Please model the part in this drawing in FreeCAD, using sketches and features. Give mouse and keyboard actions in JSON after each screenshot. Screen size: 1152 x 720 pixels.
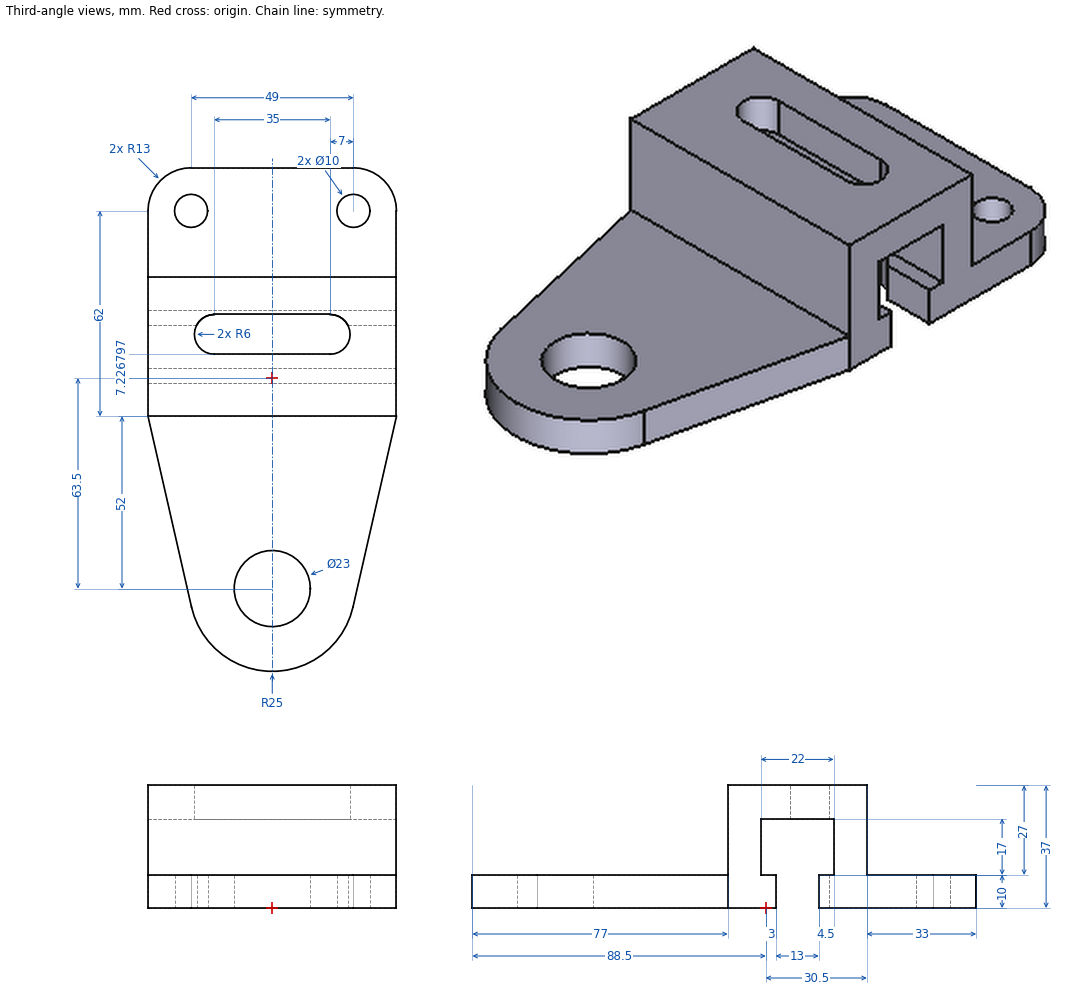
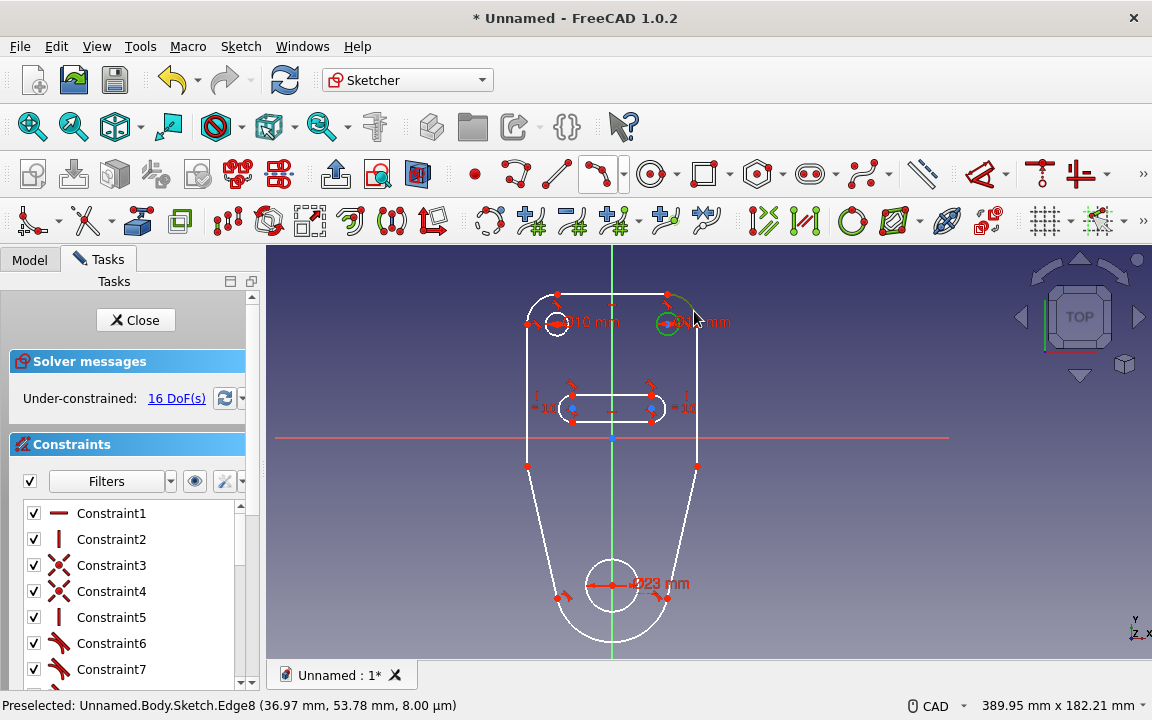
{"action": "left_click", "coordinate": [1040, 174]}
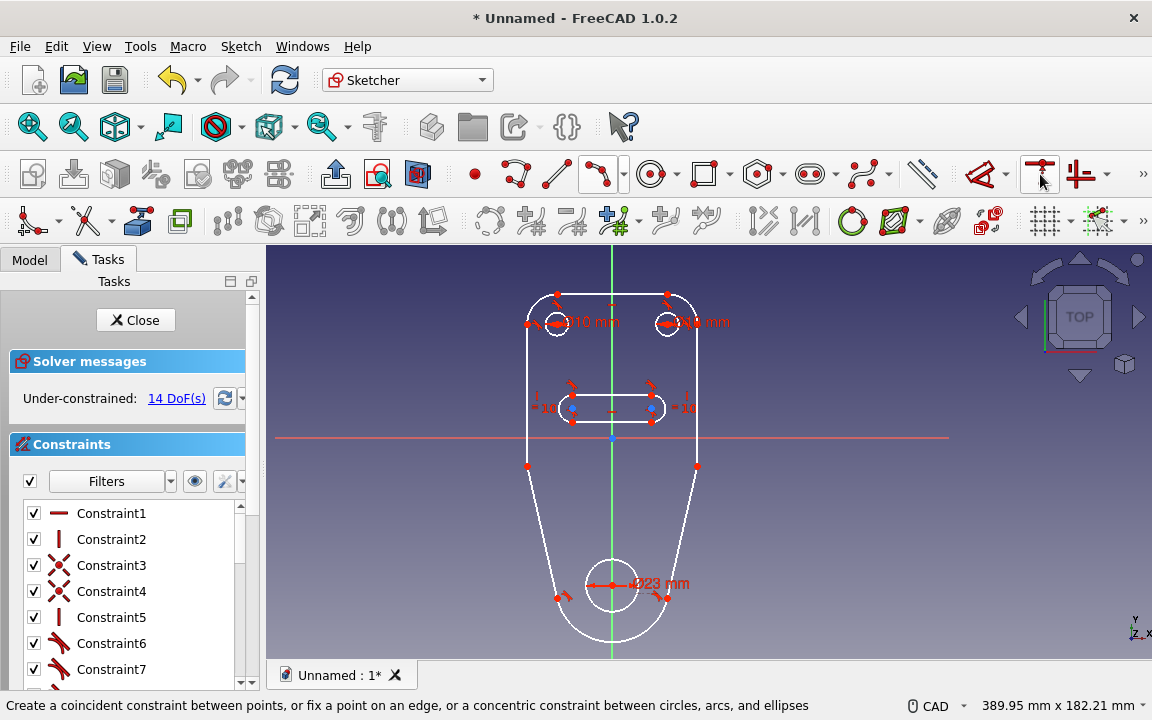
{"action": "left_click", "coordinate": [543, 298]}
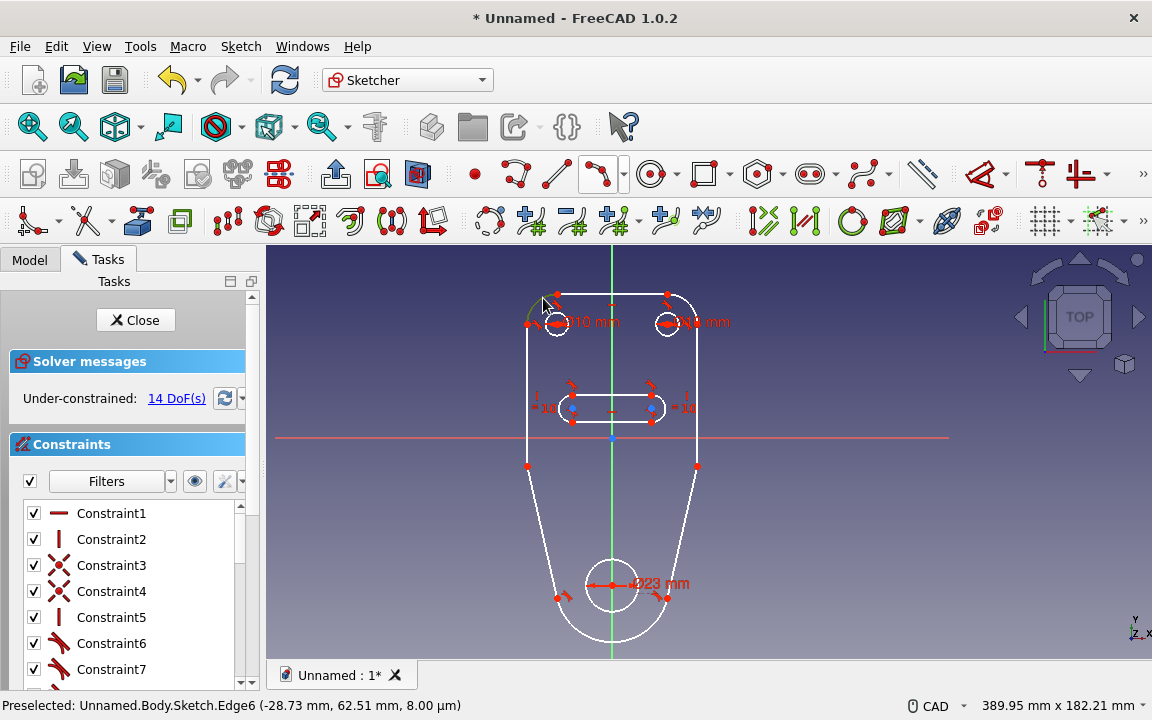
{"action": "left_click", "coordinate": [694, 311]}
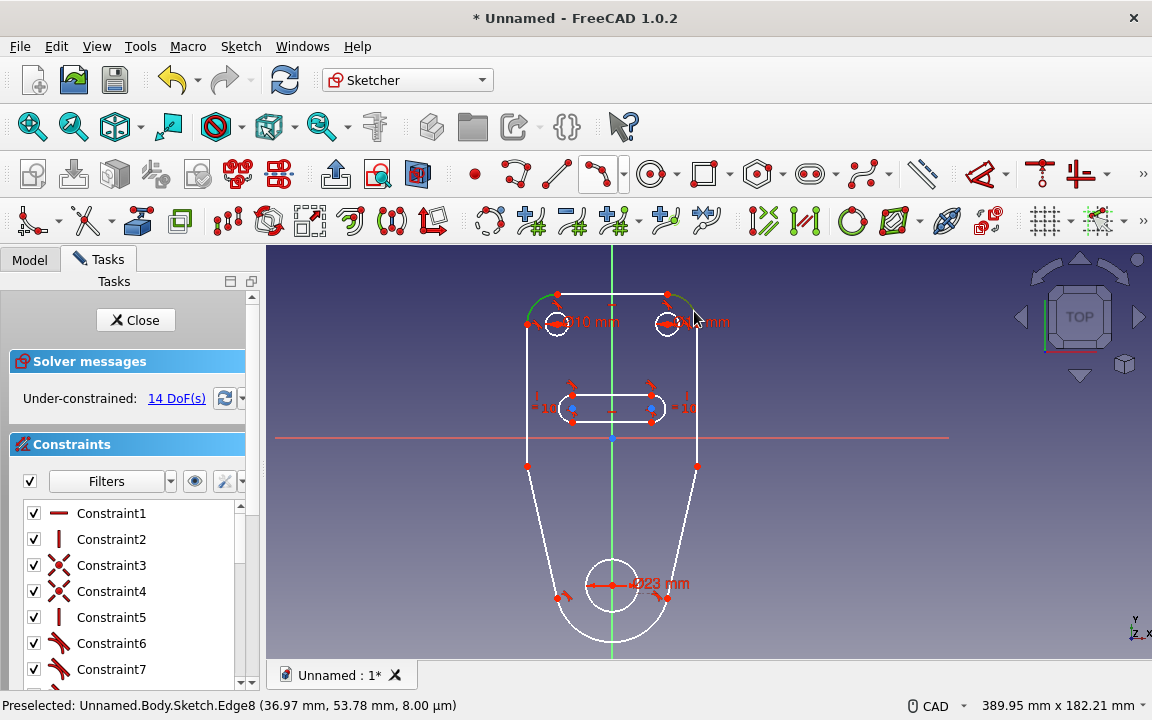
{"action": "key", "text": "e"}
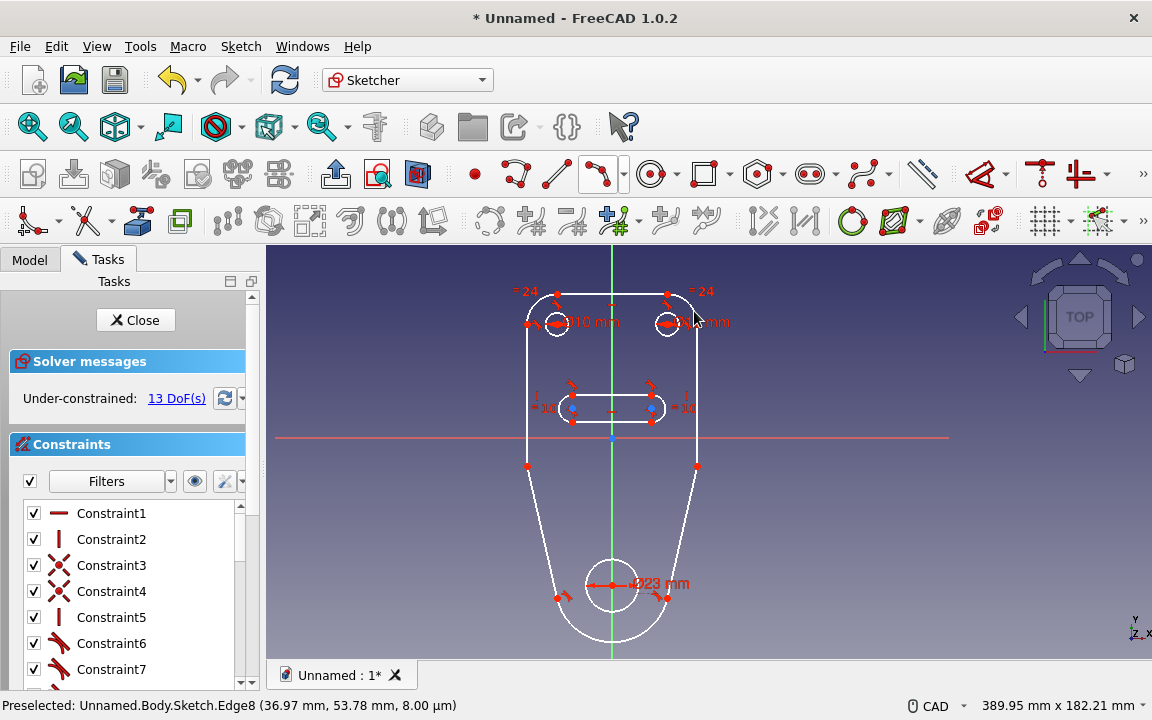
{"action": "left_click", "coordinate": [612, 586]}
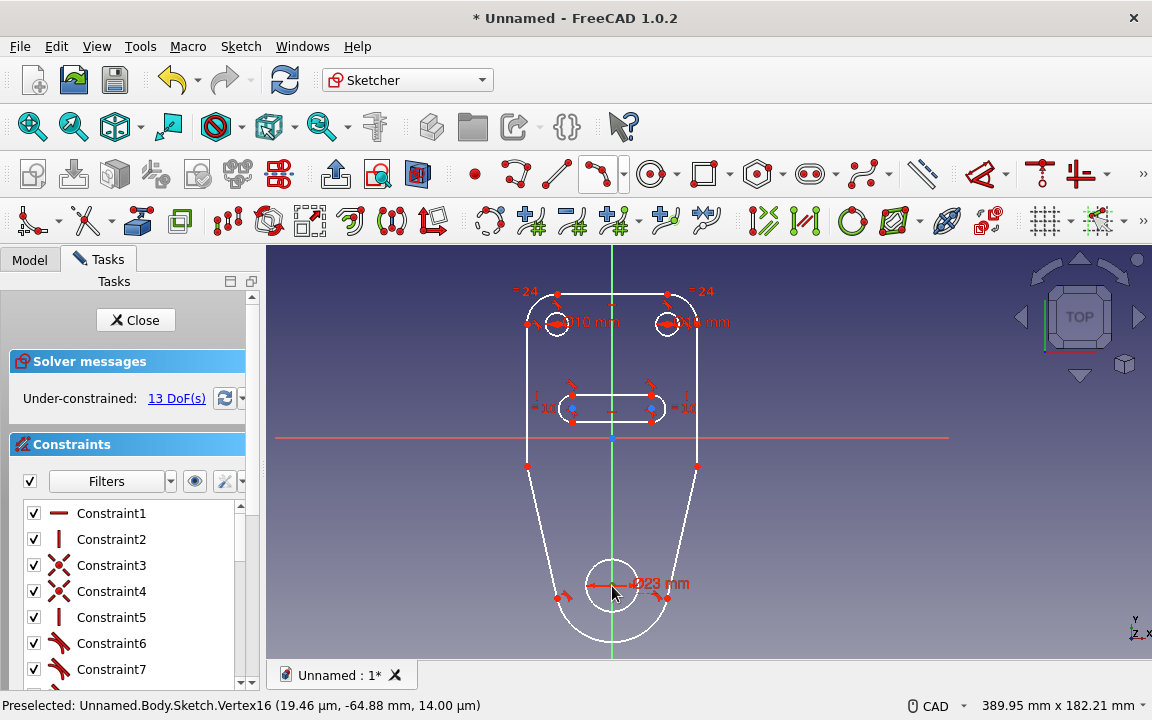
{"action": "left_click", "coordinate": [612, 529]}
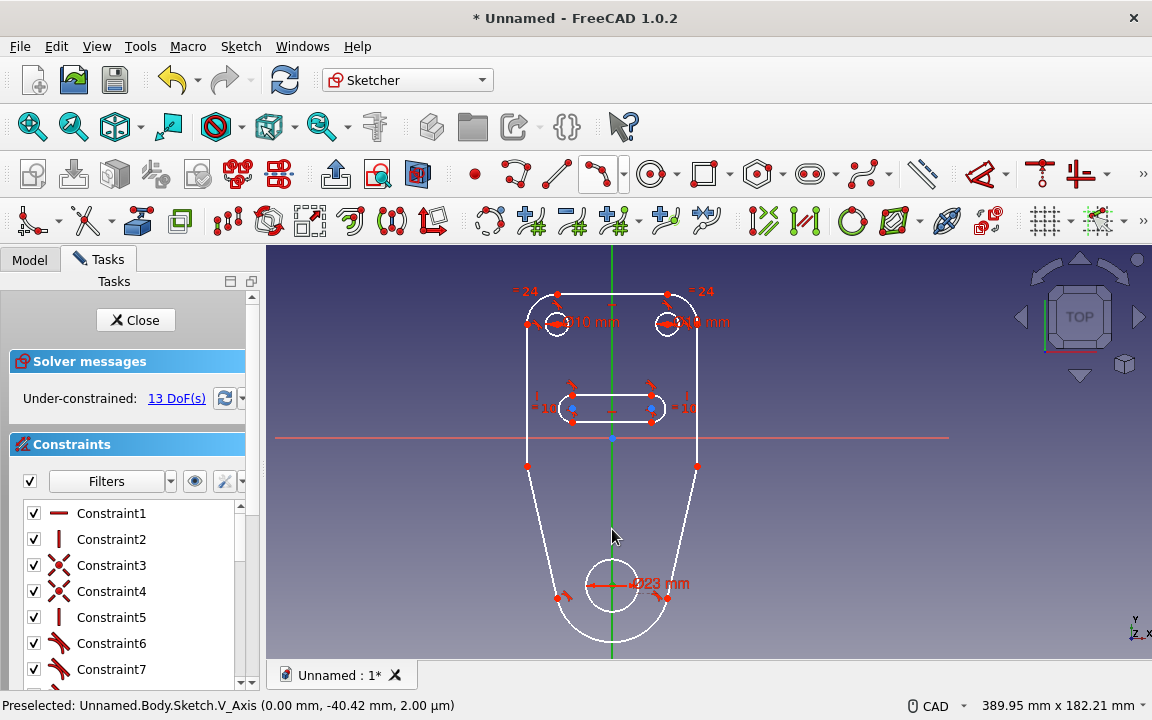
{"action": "left_click", "coordinate": [1040, 174]}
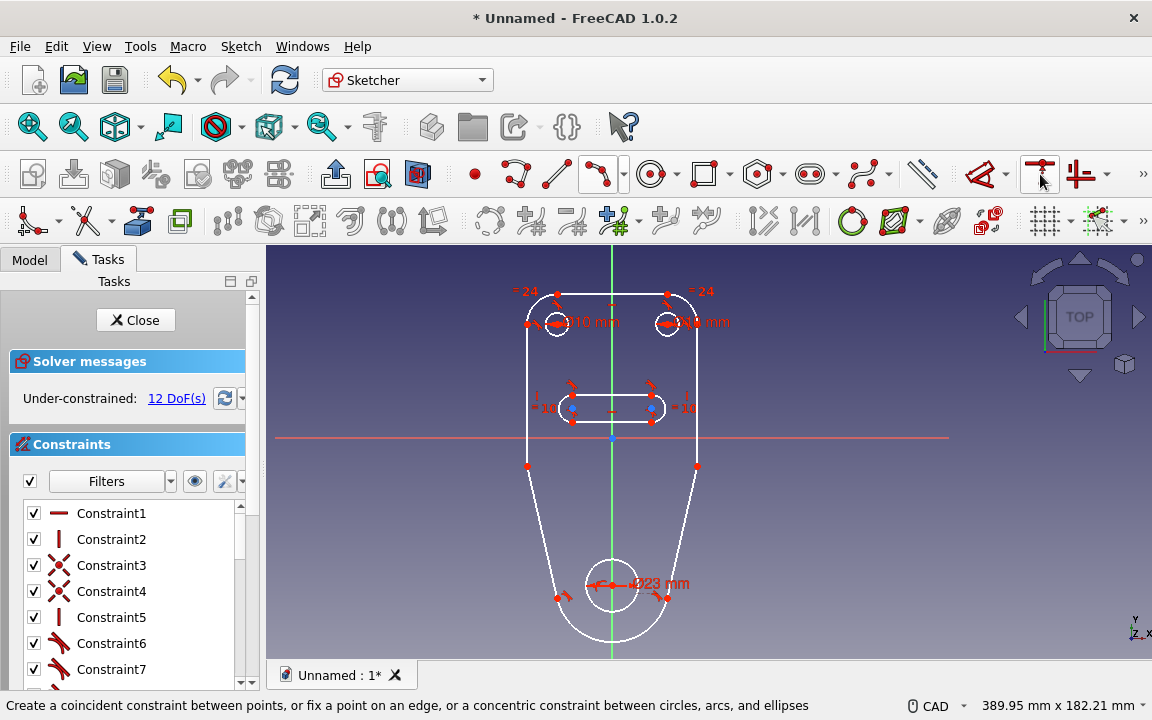
{"action": "left_click", "coordinate": [527, 466]}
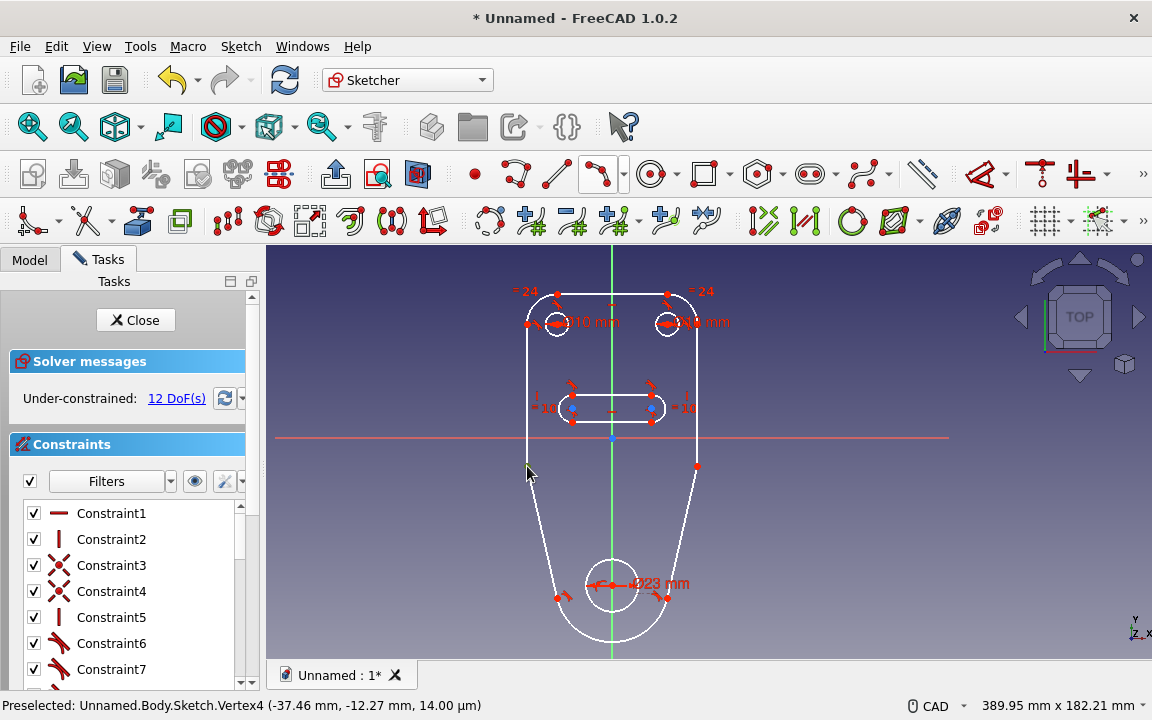
{"action": "left_click", "coordinate": [697, 466]}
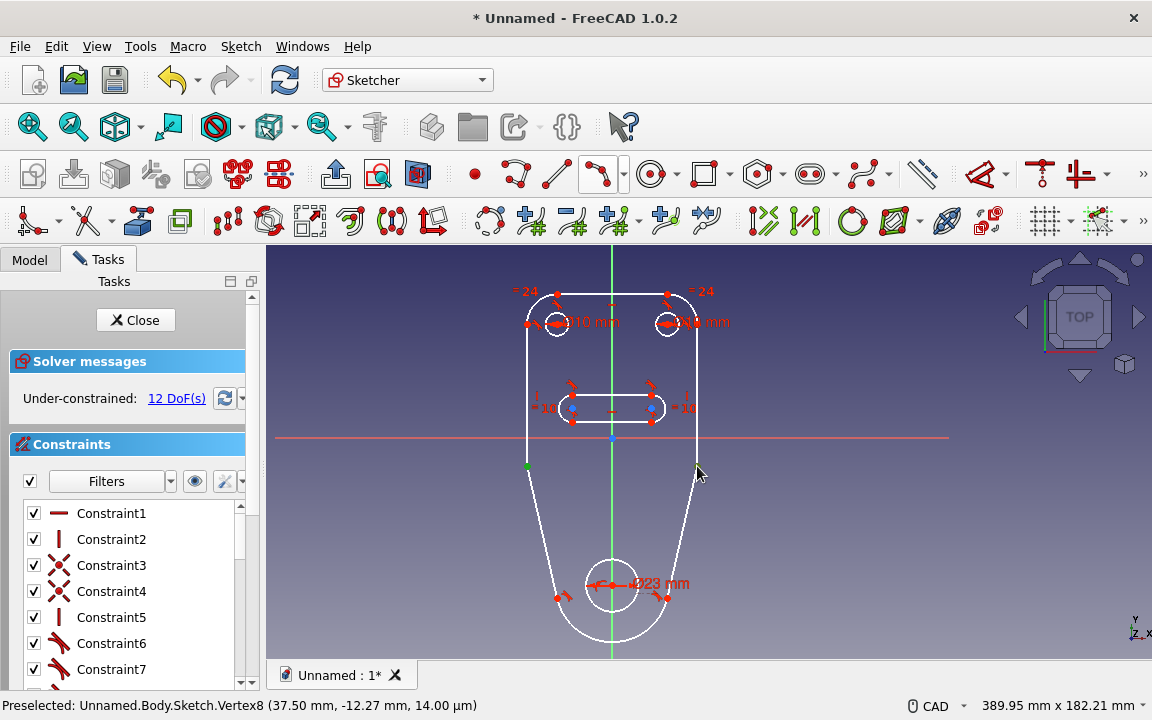
{"action": "left_click", "coordinate": [612, 529]}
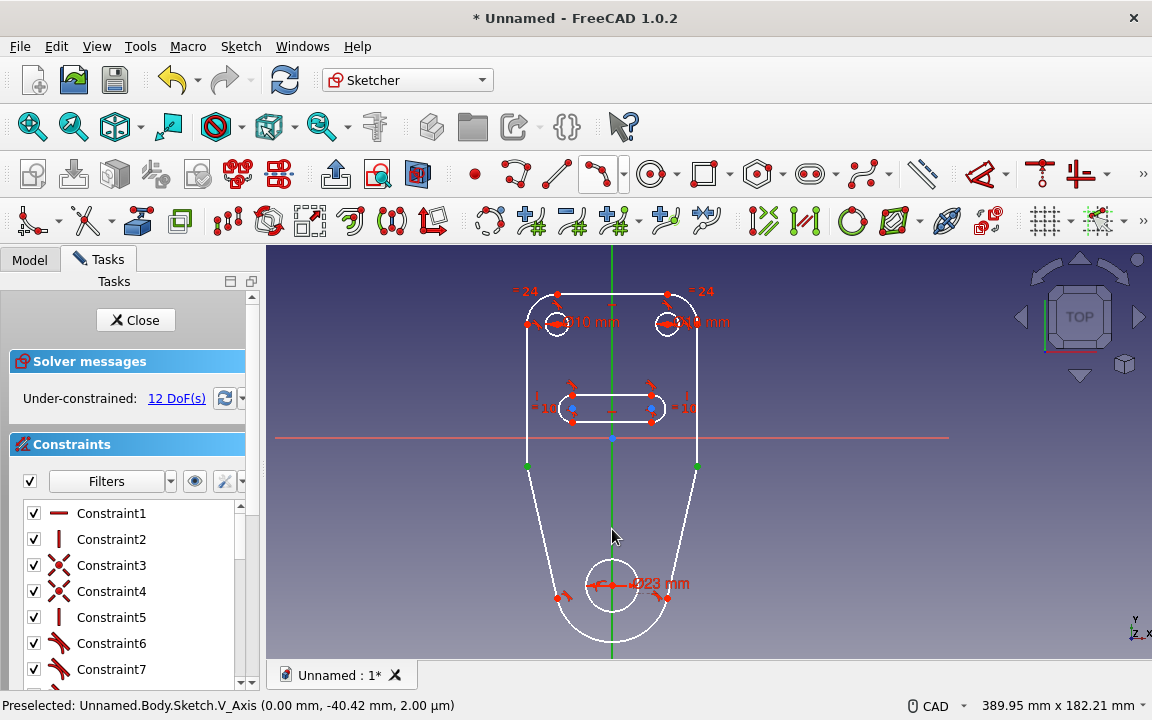
{"action": "key", "text": "s"}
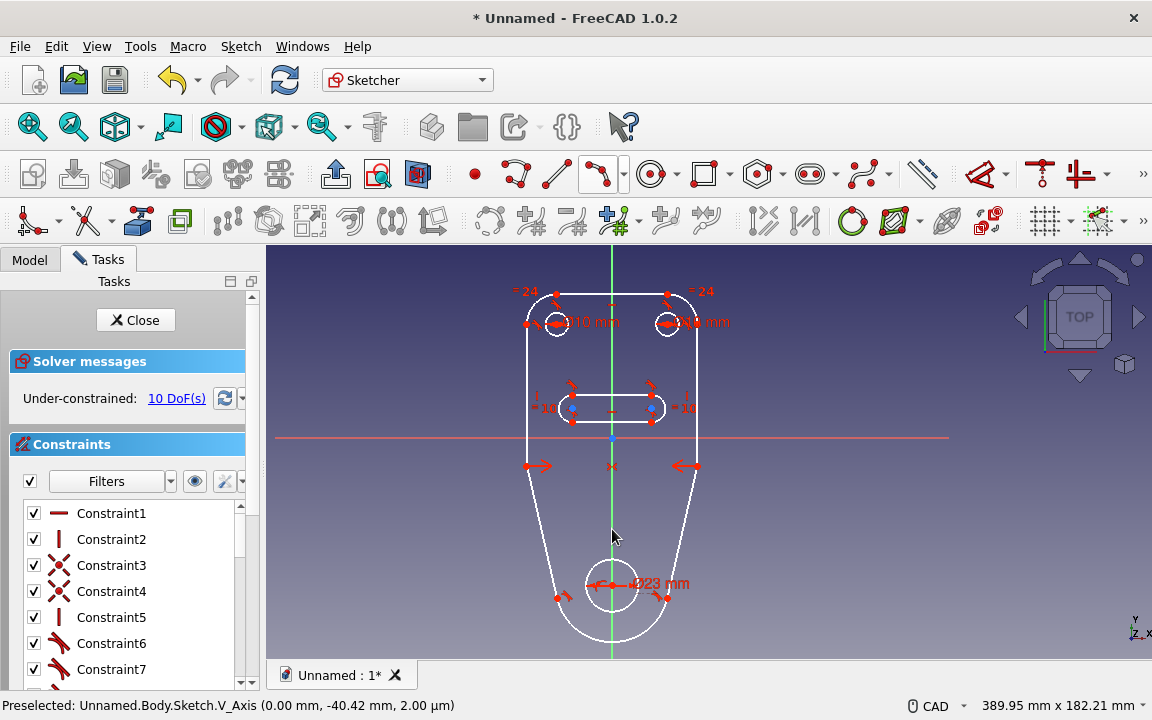
{"action": "left_click", "coordinate": [980, 174]}